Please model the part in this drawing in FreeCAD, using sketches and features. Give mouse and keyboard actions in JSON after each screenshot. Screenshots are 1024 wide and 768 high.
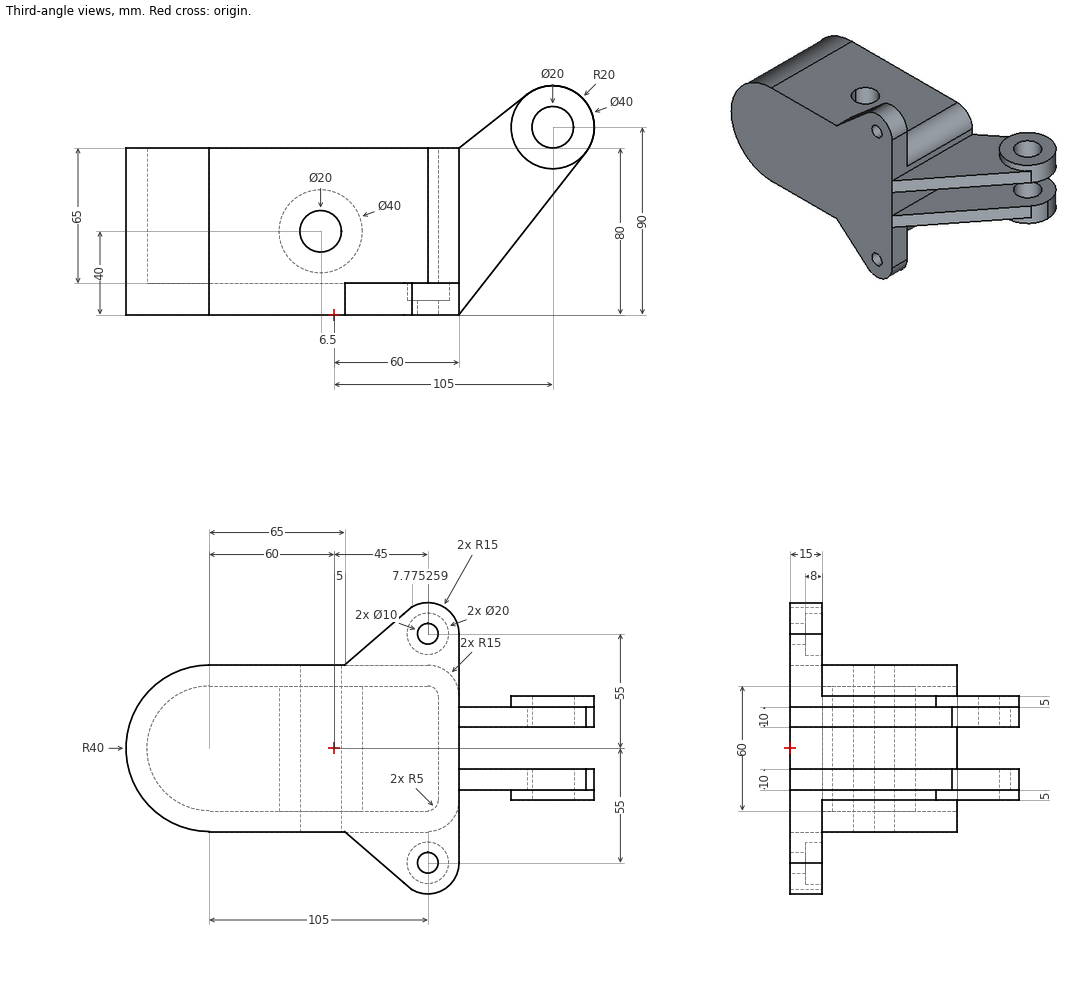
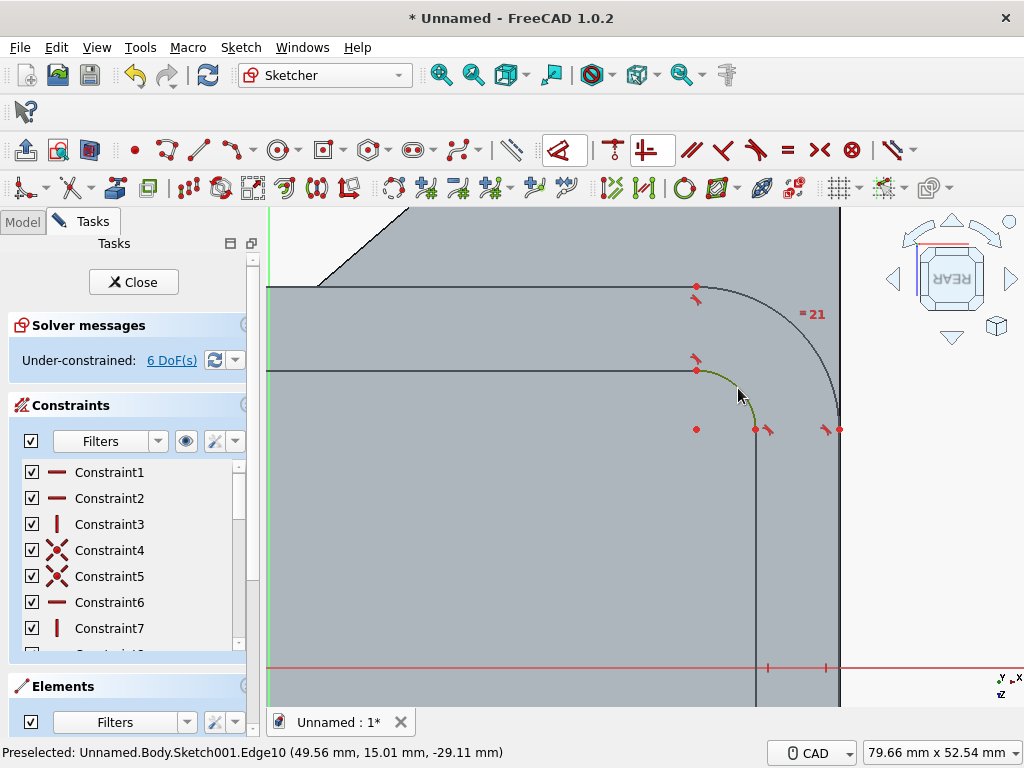
{"action": "left_click", "coordinate": [582, 150]}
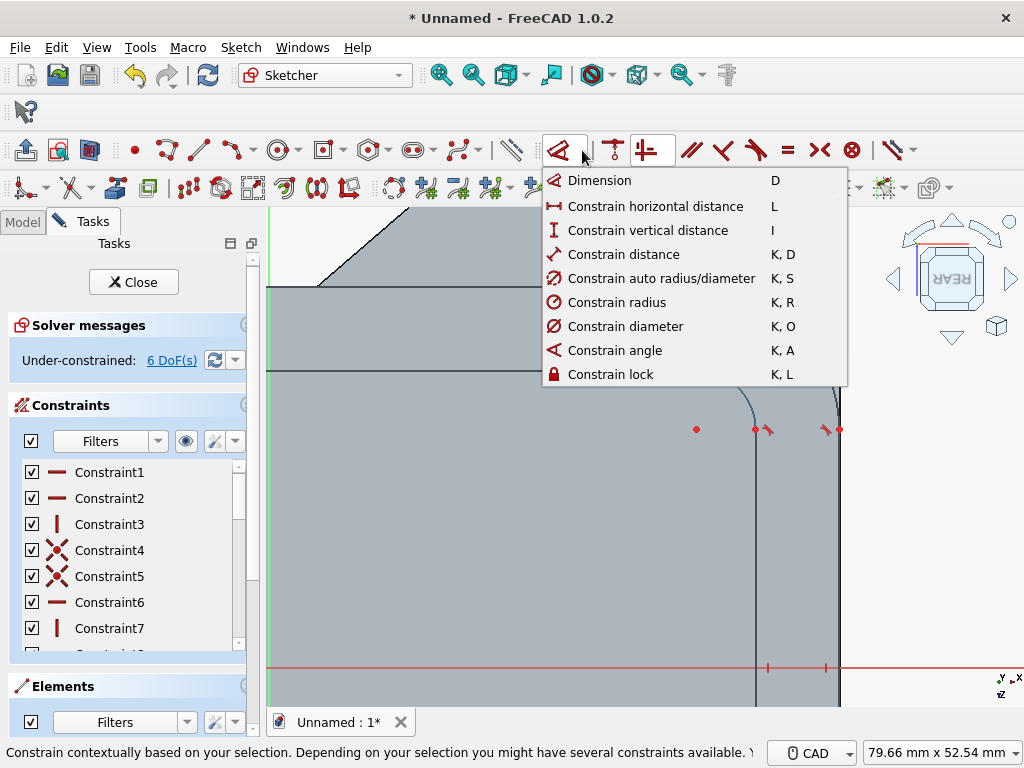
{"action": "left_click", "coordinate": [695, 302]}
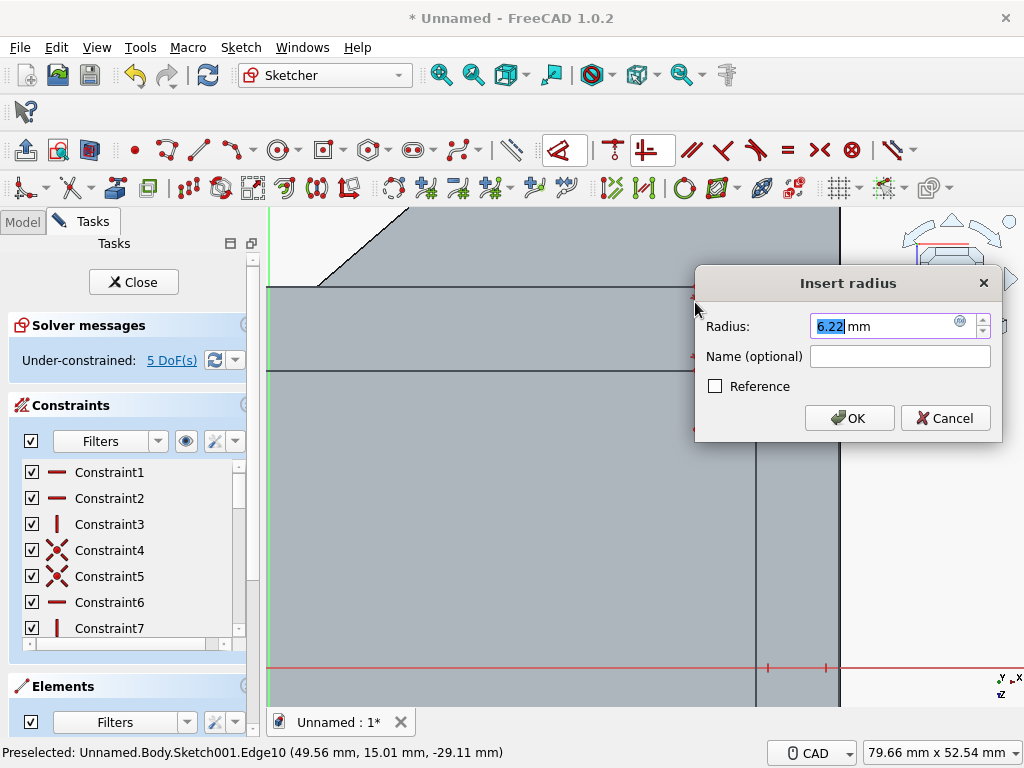
{"action": "type", "text": "5"}
{"action": "key", "text": "Return"}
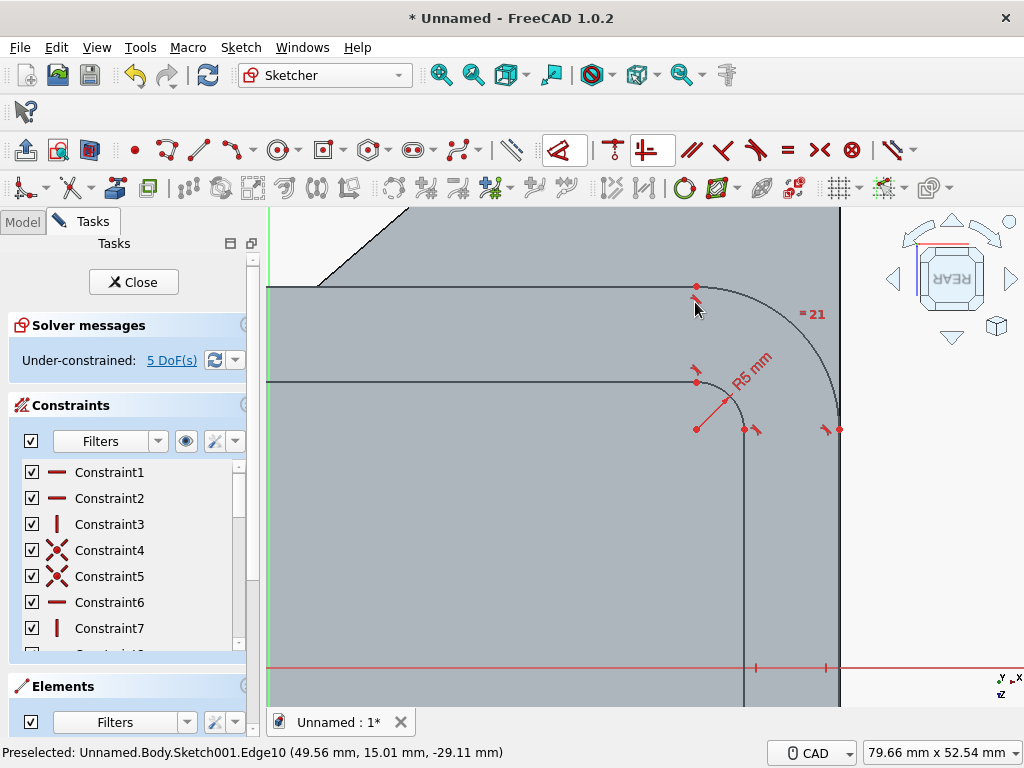
{"action": "scroll", "coordinate": [739, 388], "scroll_direction": "down", "scroll_amount": 7}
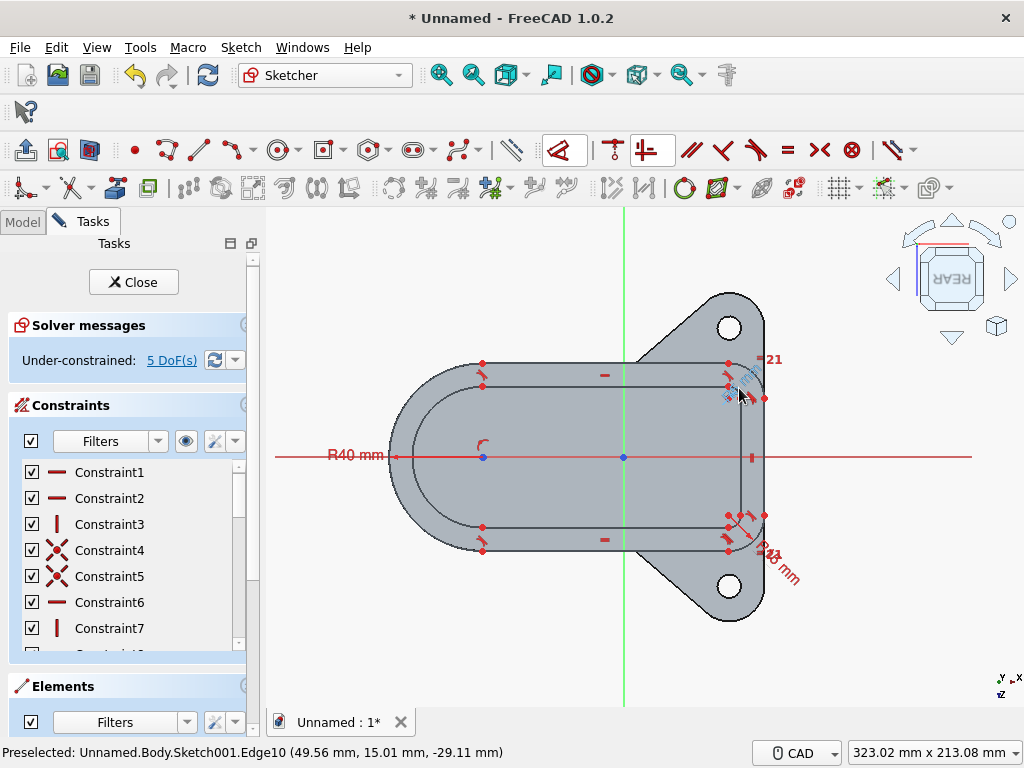
{"action": "left_click", "coordinate": [655, 363]}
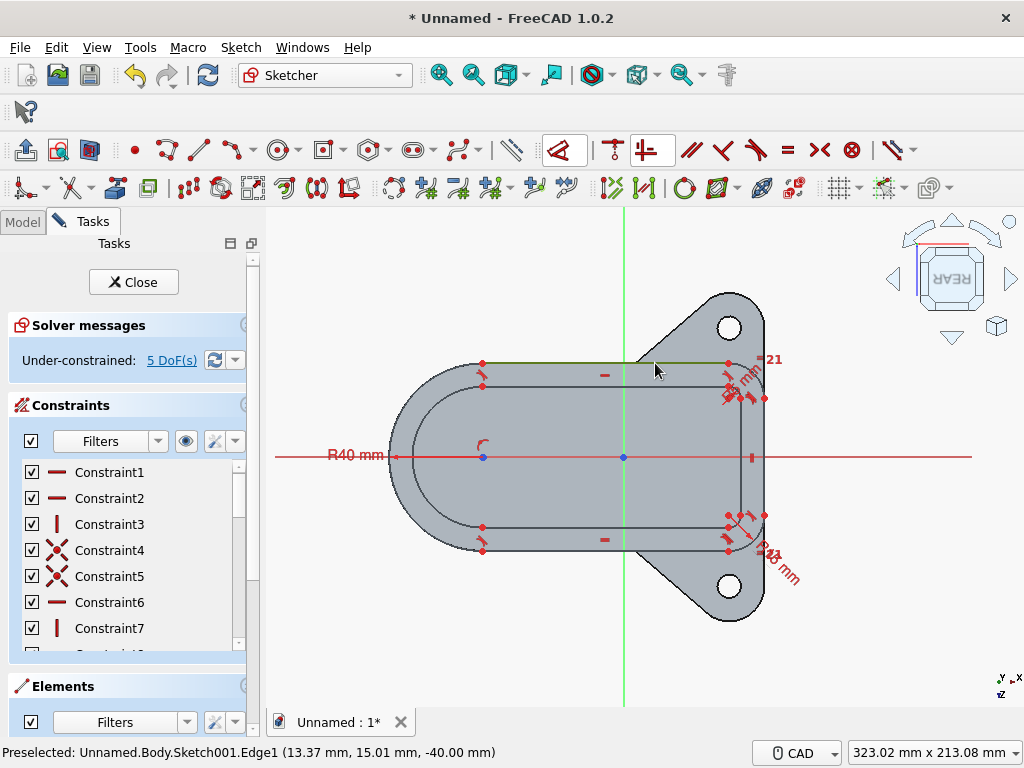
{"action": "left_click", "coordinate": [582, 150]}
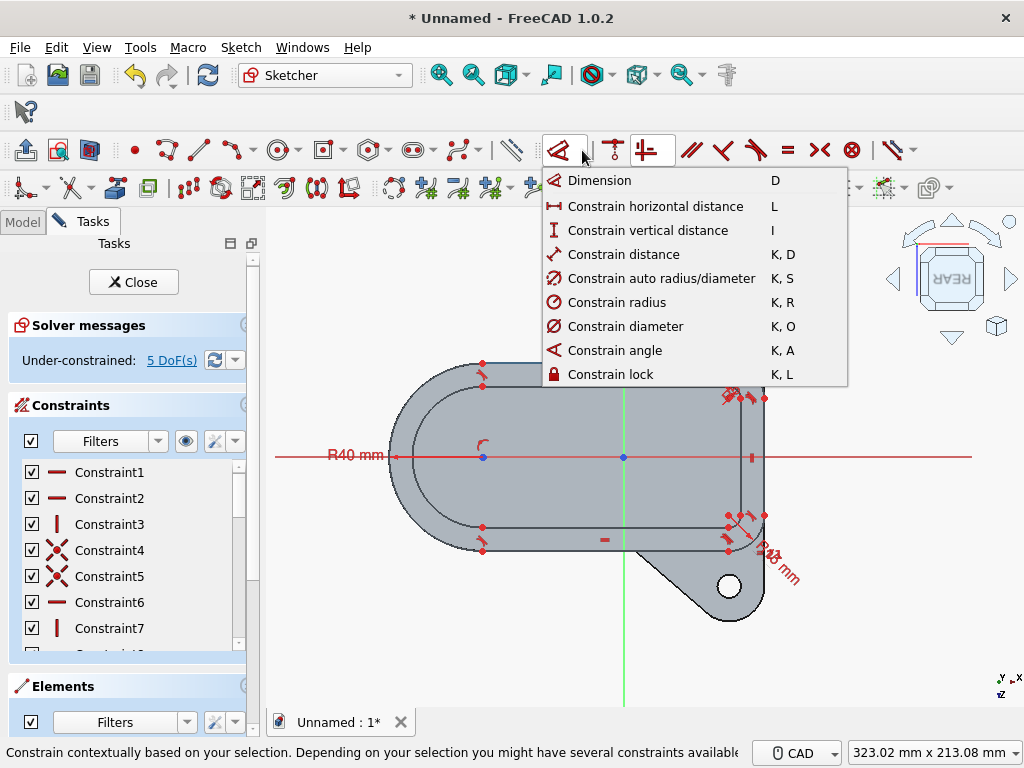
{"action": "left_click", "coordinate": [695, 206]}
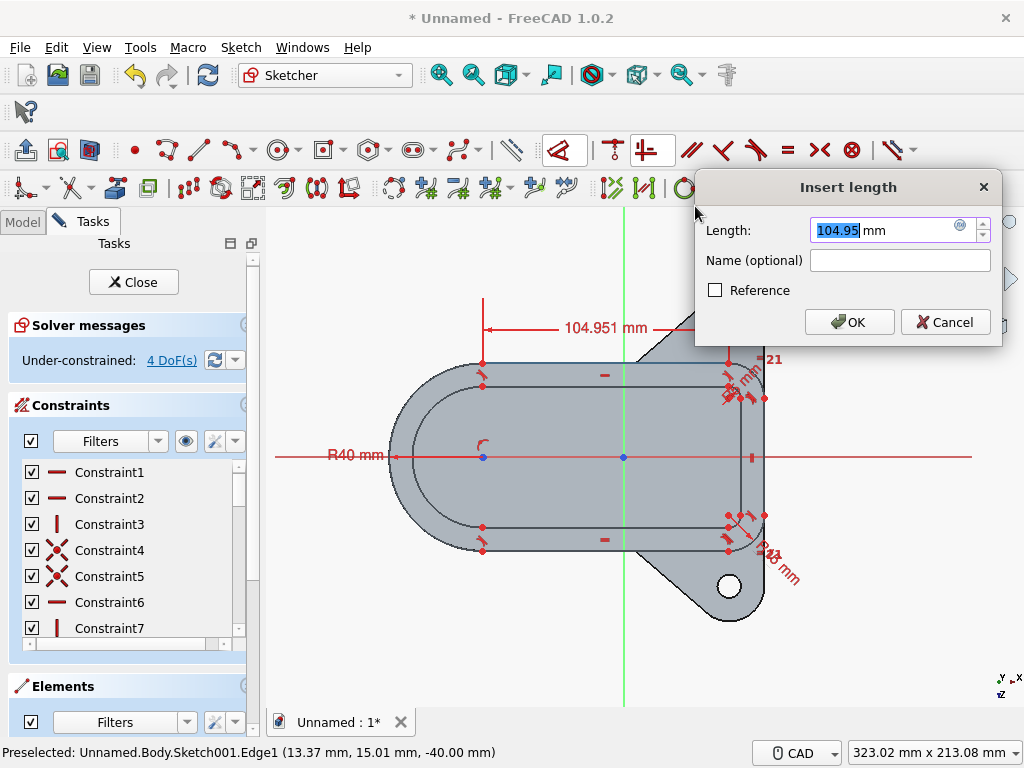
{"action": "type", "text": "105"}
{"action": "key", "text": "Return"}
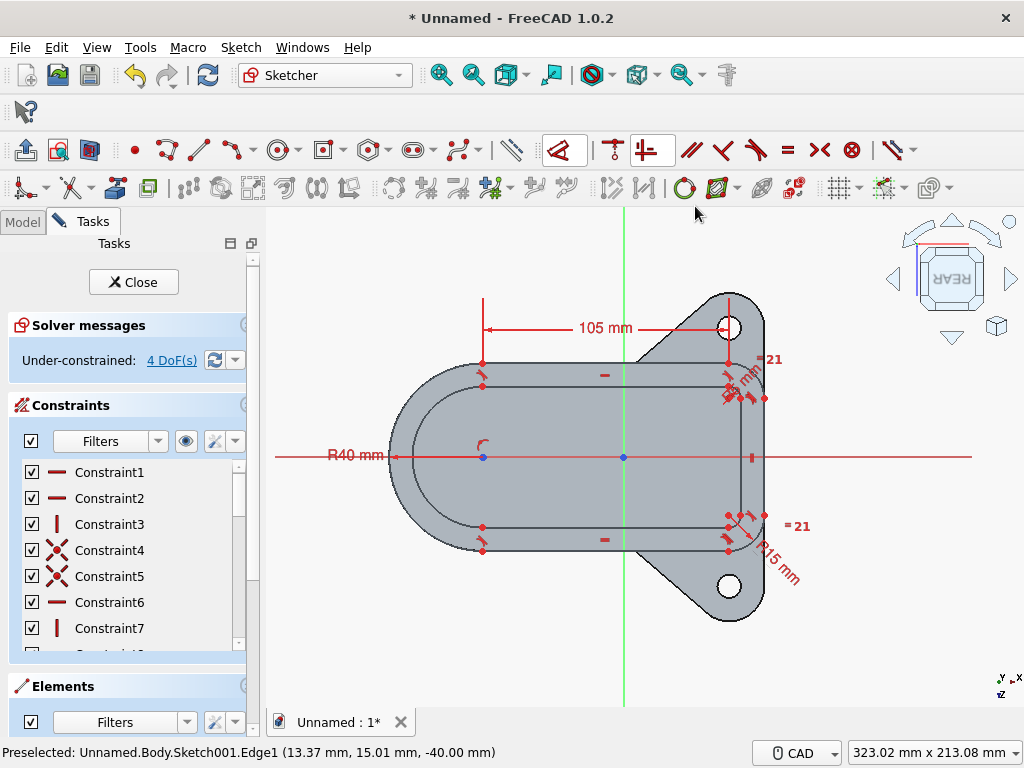
{"action": "left_click", "coordinate": [557, 551]}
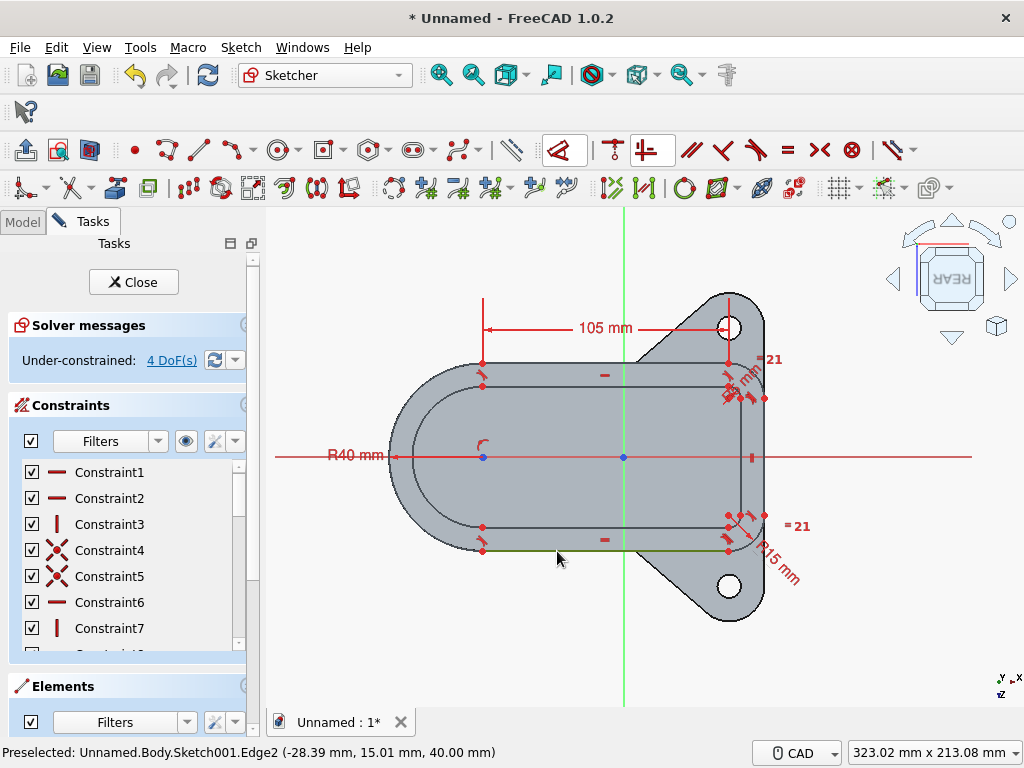
{"action": "key", "text": "l"}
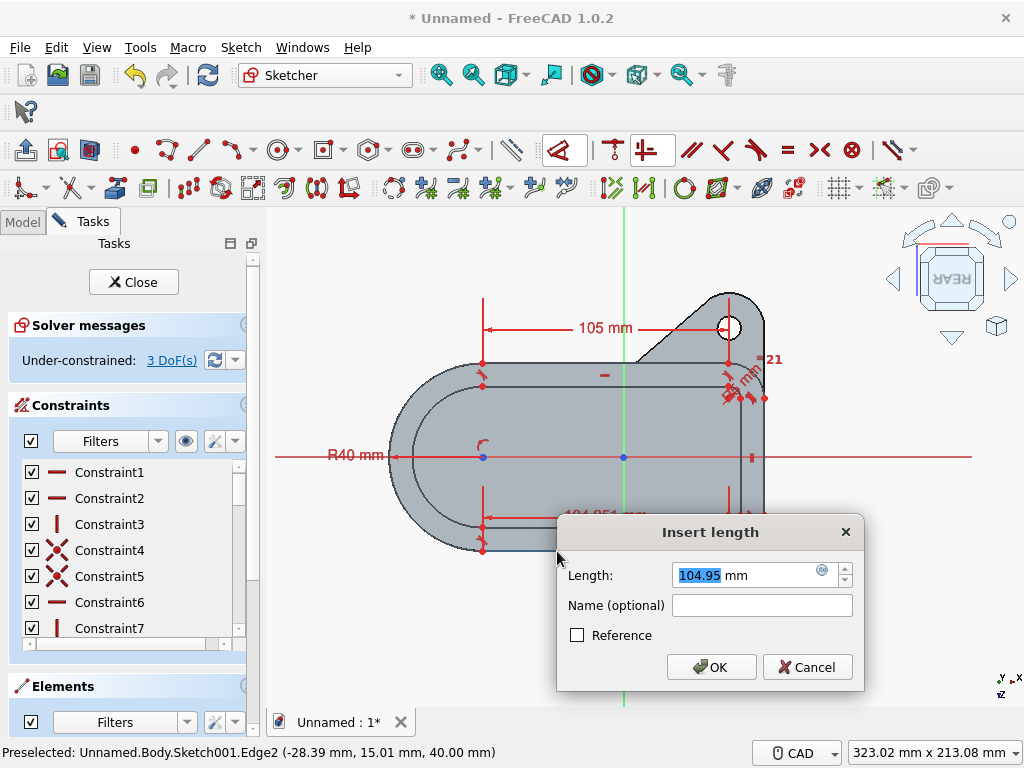
{"action": "type", "text": "105"}
{"action": "key", "text": "Return"}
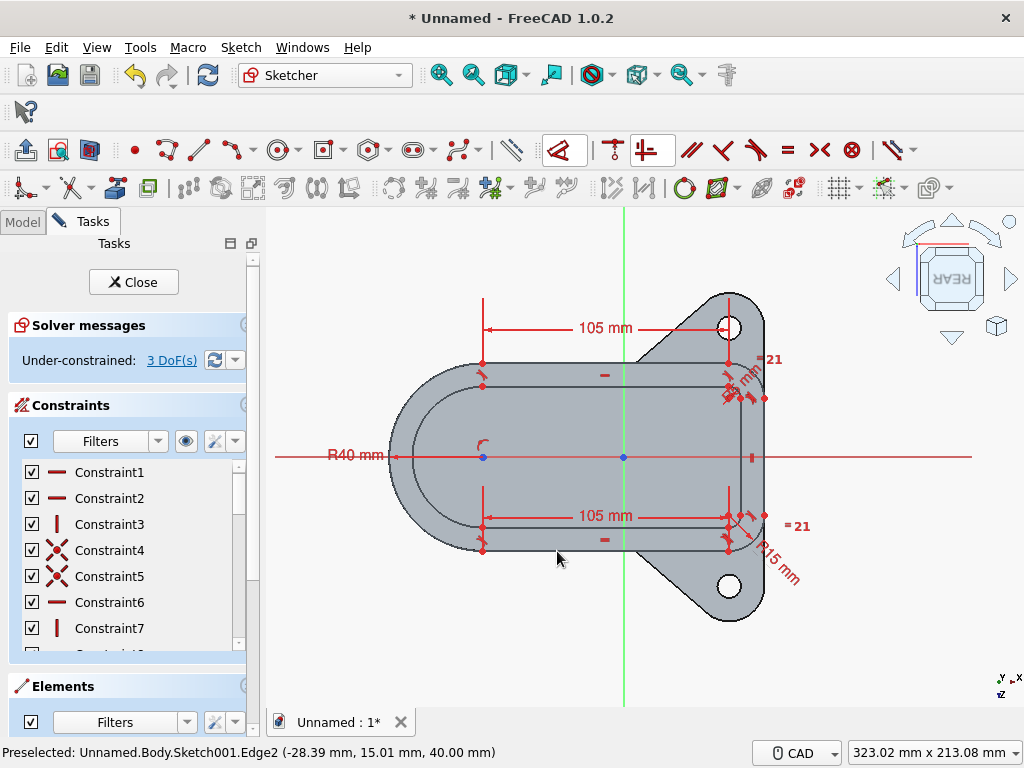
{"action": "left_click", "coordinate": [557, 387]}